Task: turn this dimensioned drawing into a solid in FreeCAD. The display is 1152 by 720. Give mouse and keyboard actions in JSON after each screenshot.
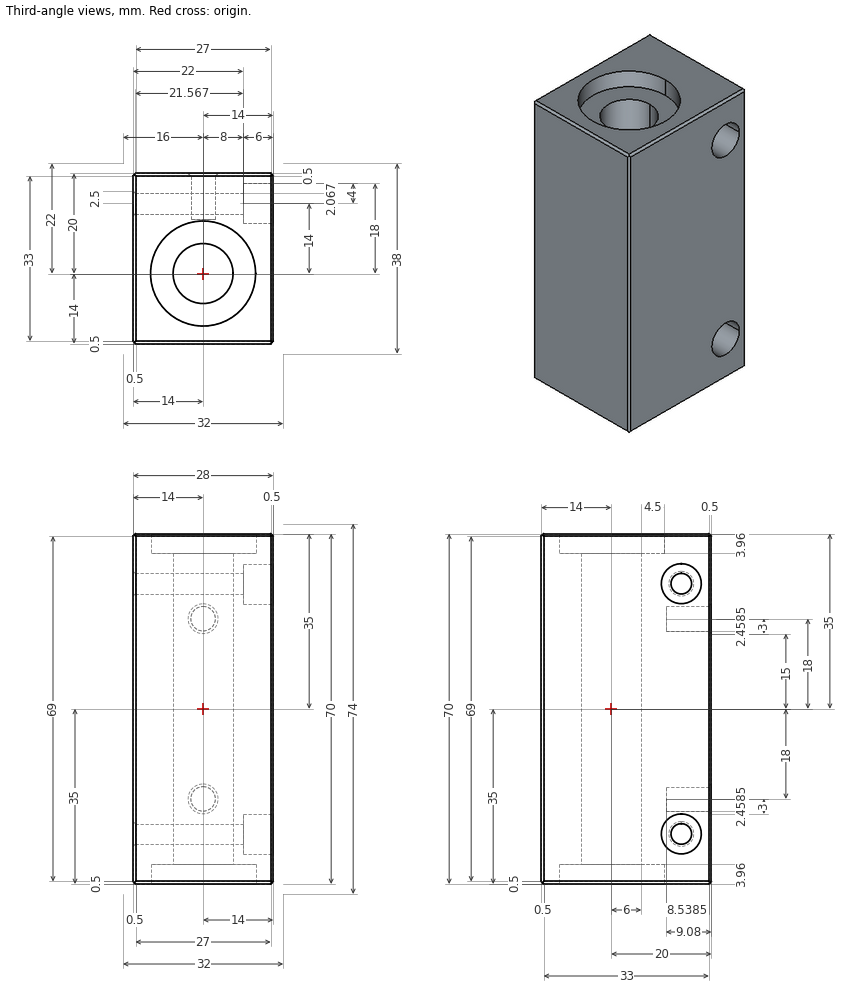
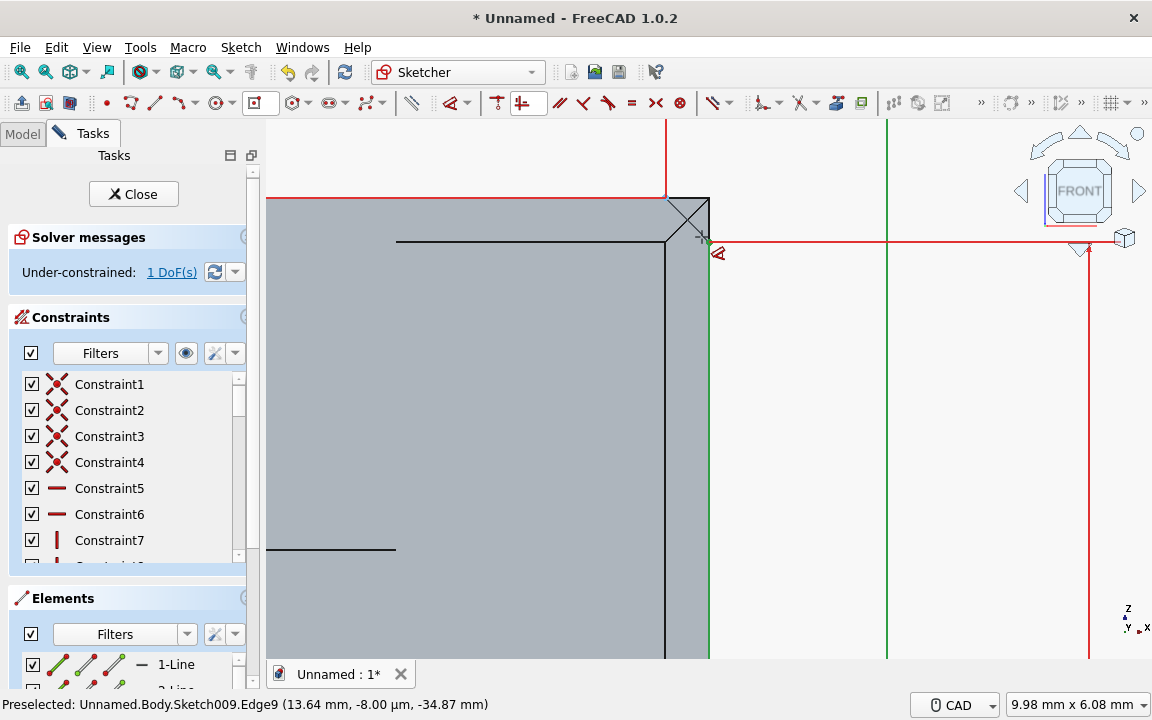
{"action": "left_click", "coordinate": [696, 229]}
{"action": "left_click", "coordinate": [687, 164]}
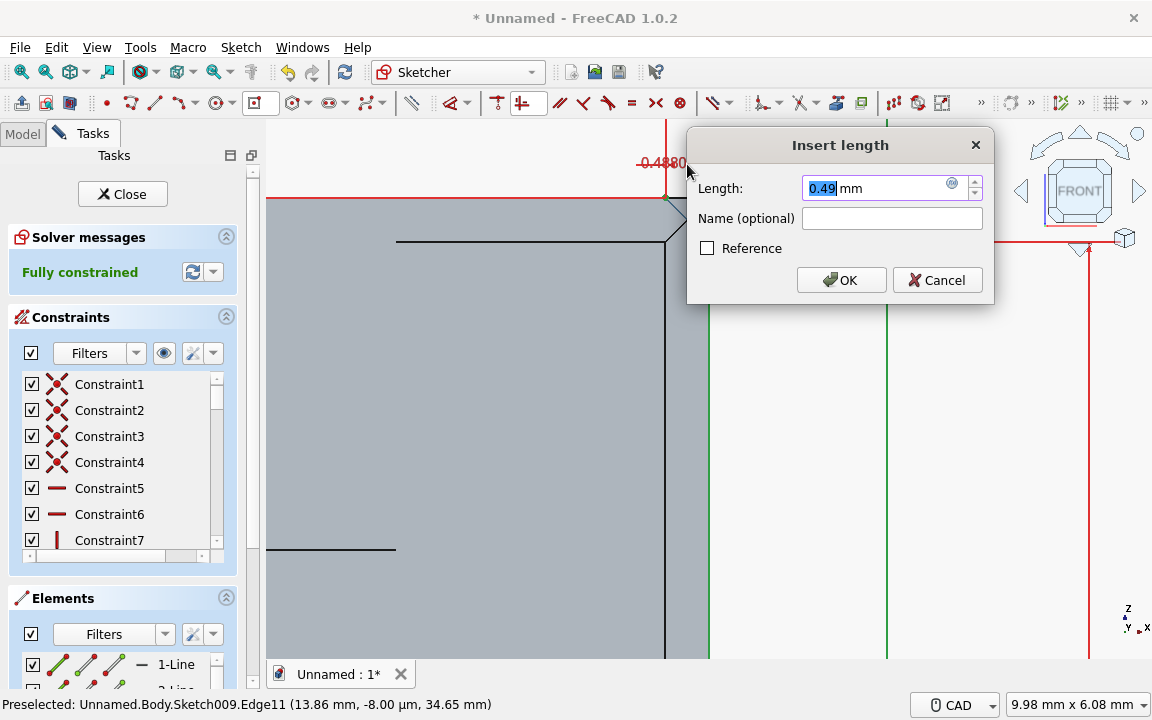
{"action": "type", "text": "0.5"}
{"action": "key", "text": "Return"}
{"action": "key", "text": "Escape"}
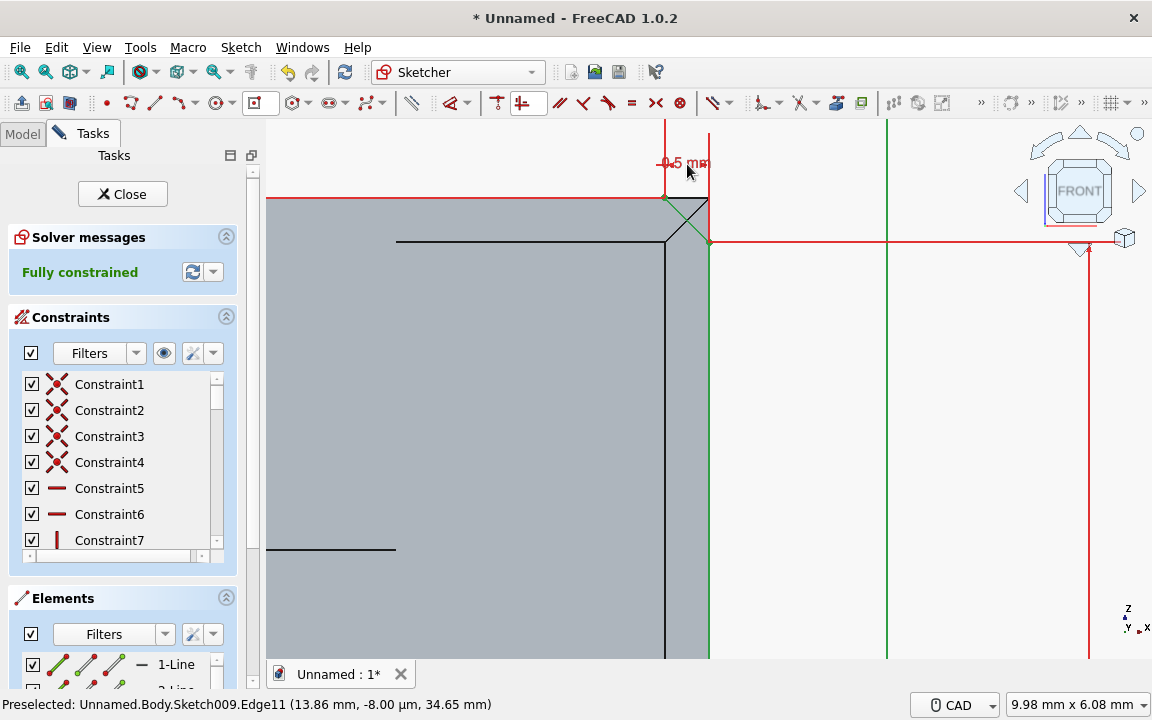
{"action": "left_click", "coordinate": [123, 194]}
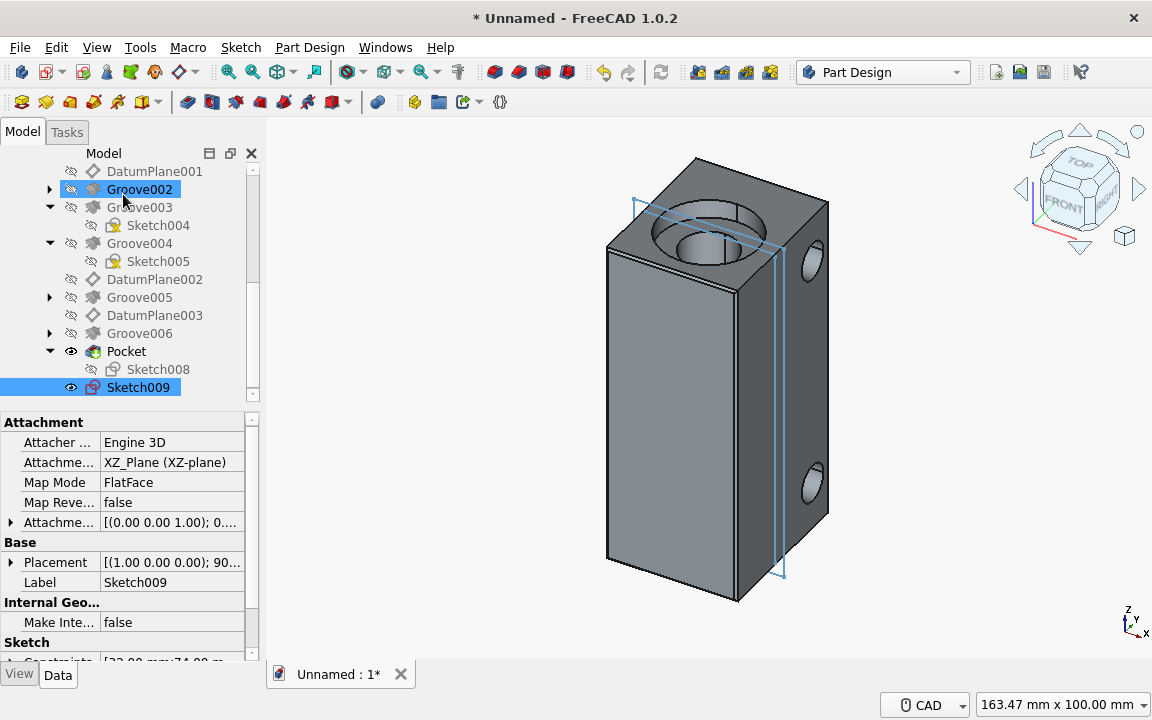
{"action": "left_click", "coordinate": [188, 102]}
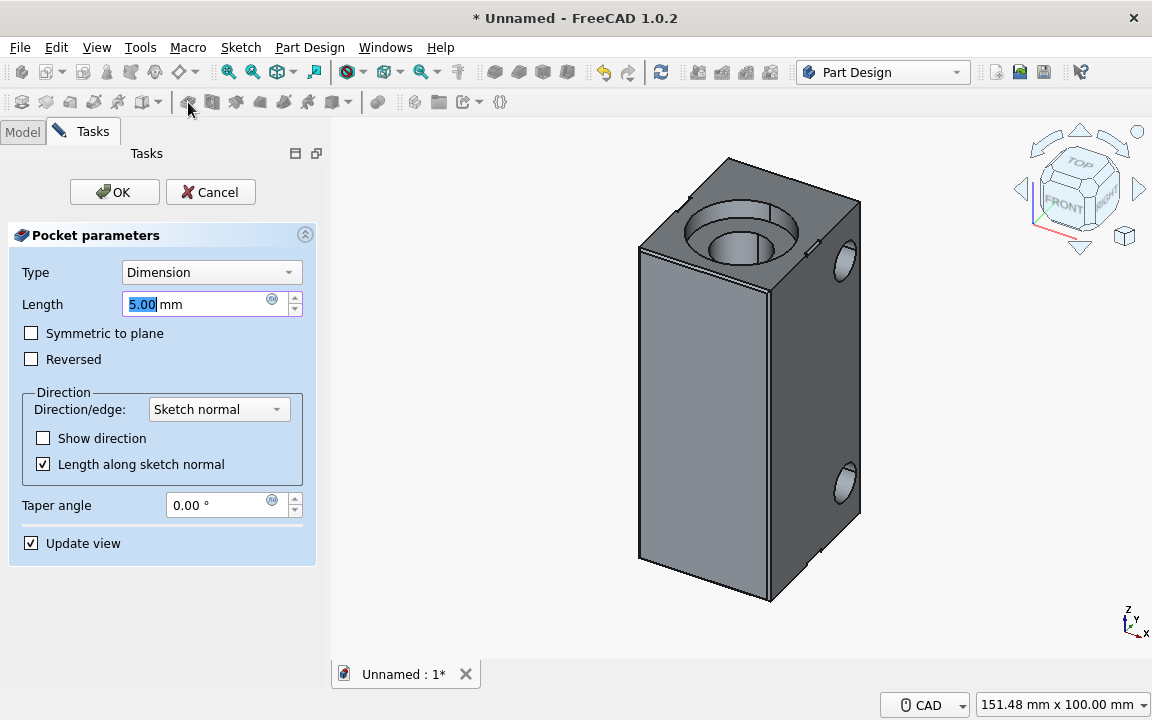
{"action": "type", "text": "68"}
{"action": "key", "text": "Tab"}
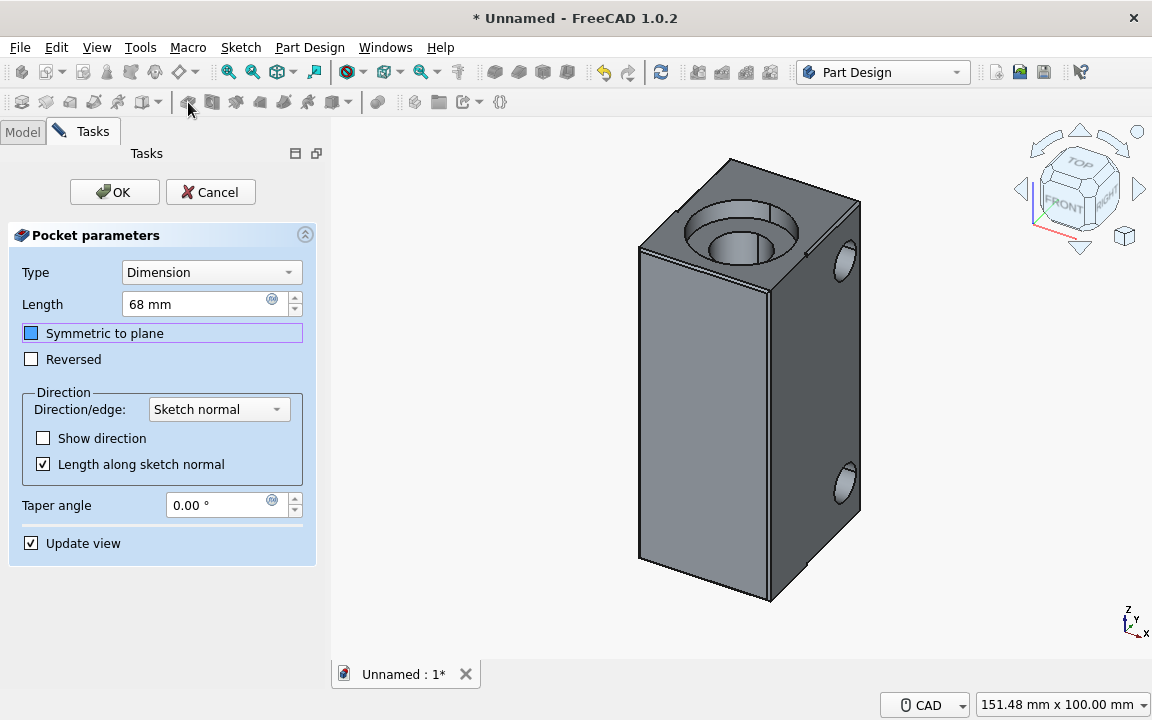
{"action": "left_click", "coordinate": [30, 333]}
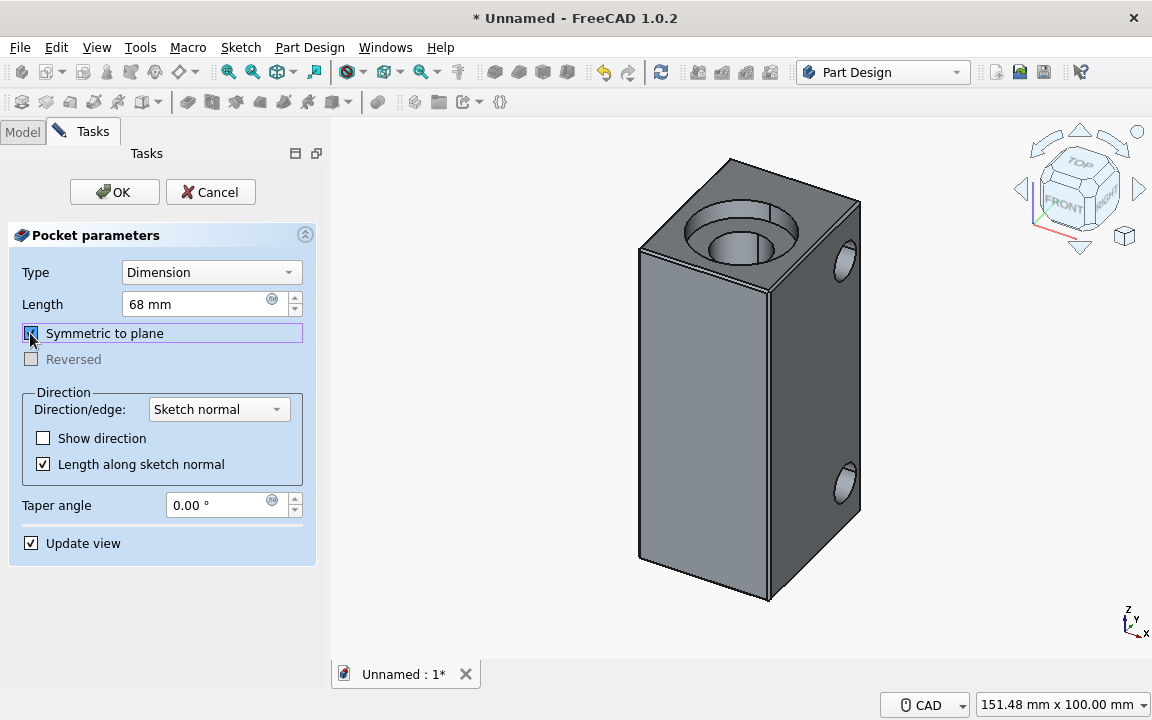
{"action": "left_click", "coordinate": [115, 192]}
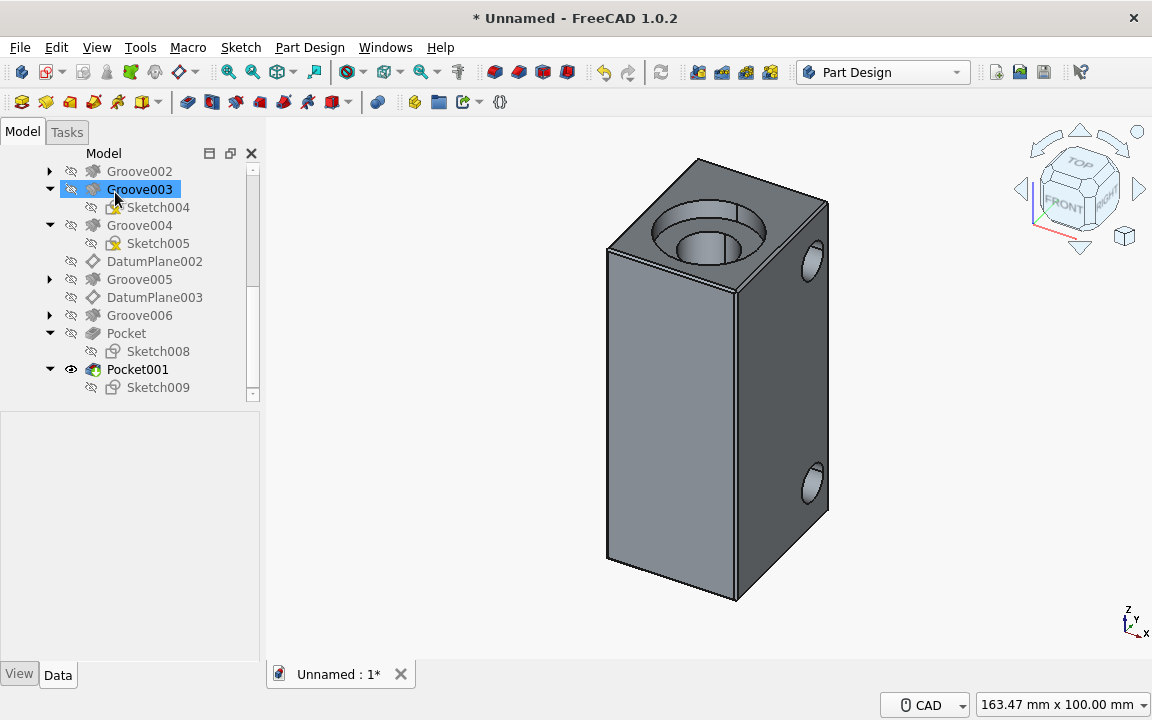
{"action": "key", "text": "0"}